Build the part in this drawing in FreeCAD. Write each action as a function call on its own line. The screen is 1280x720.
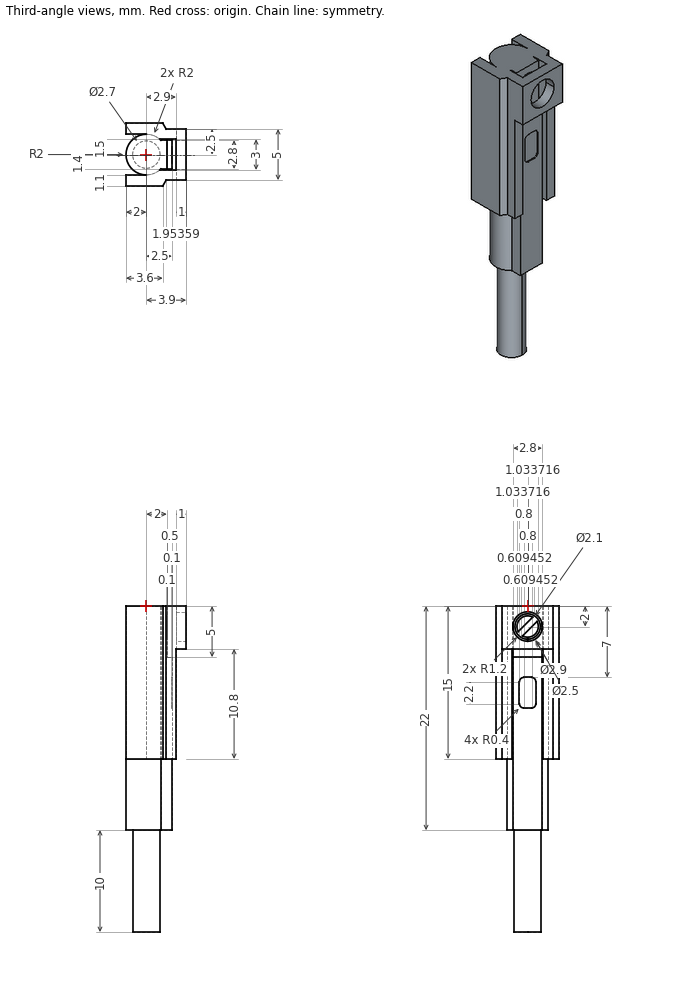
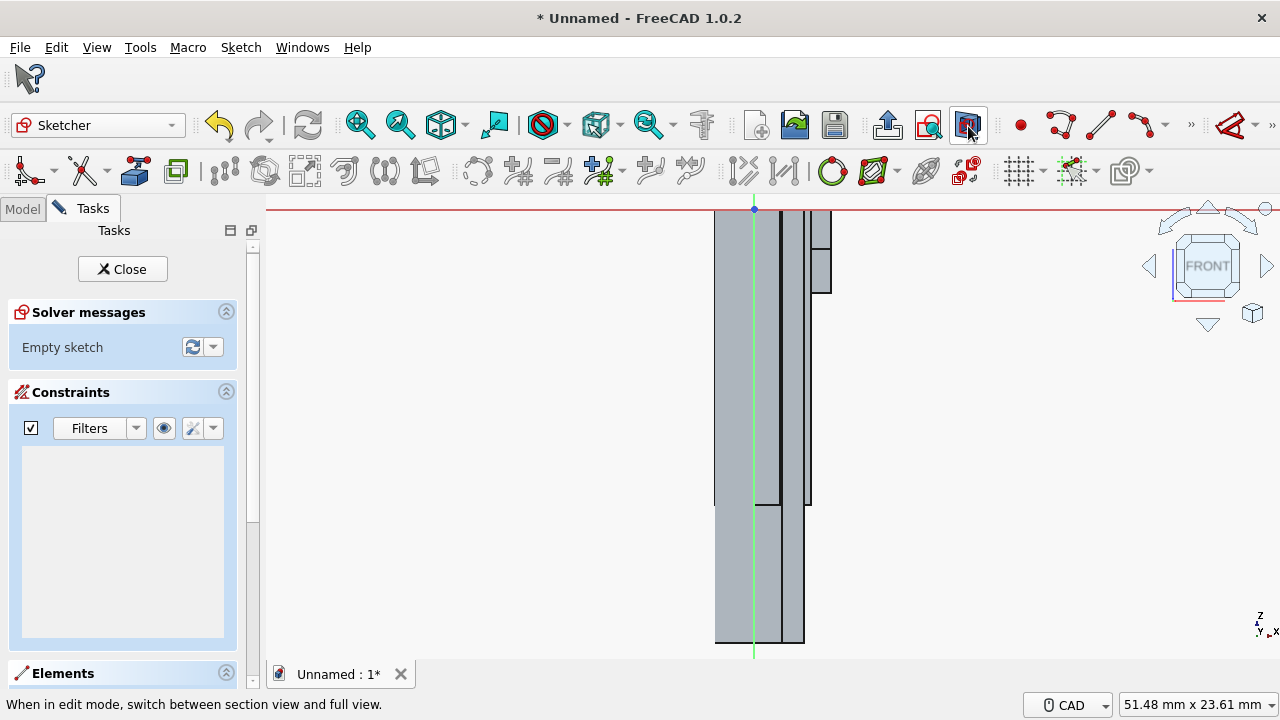
scroll(704, 426, down, 5)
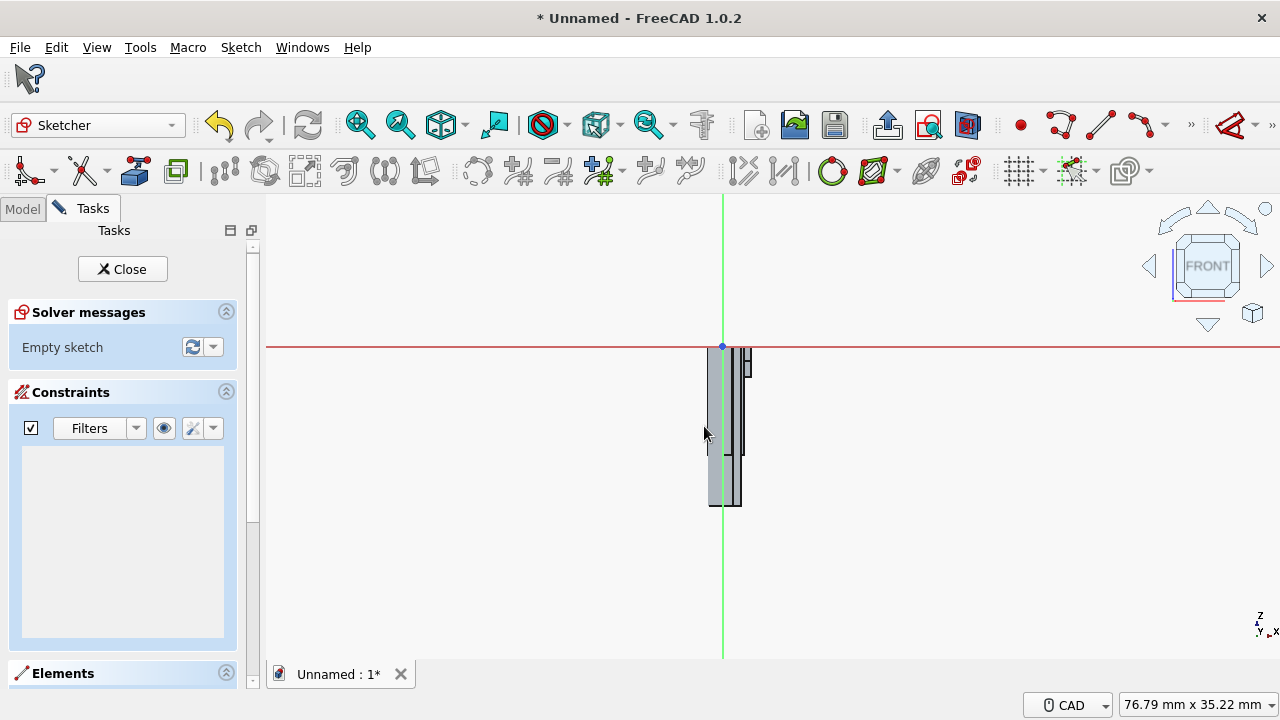
scroll(736, 355, up, 10)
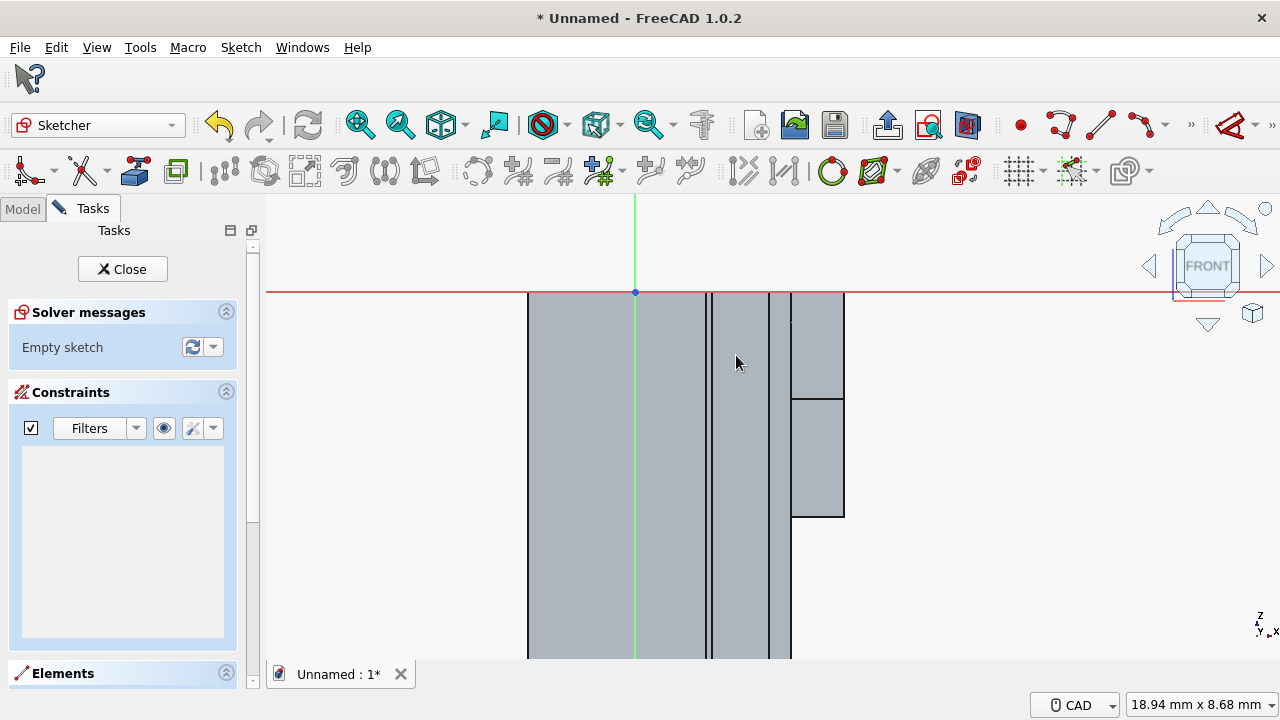
key(g)
key(r)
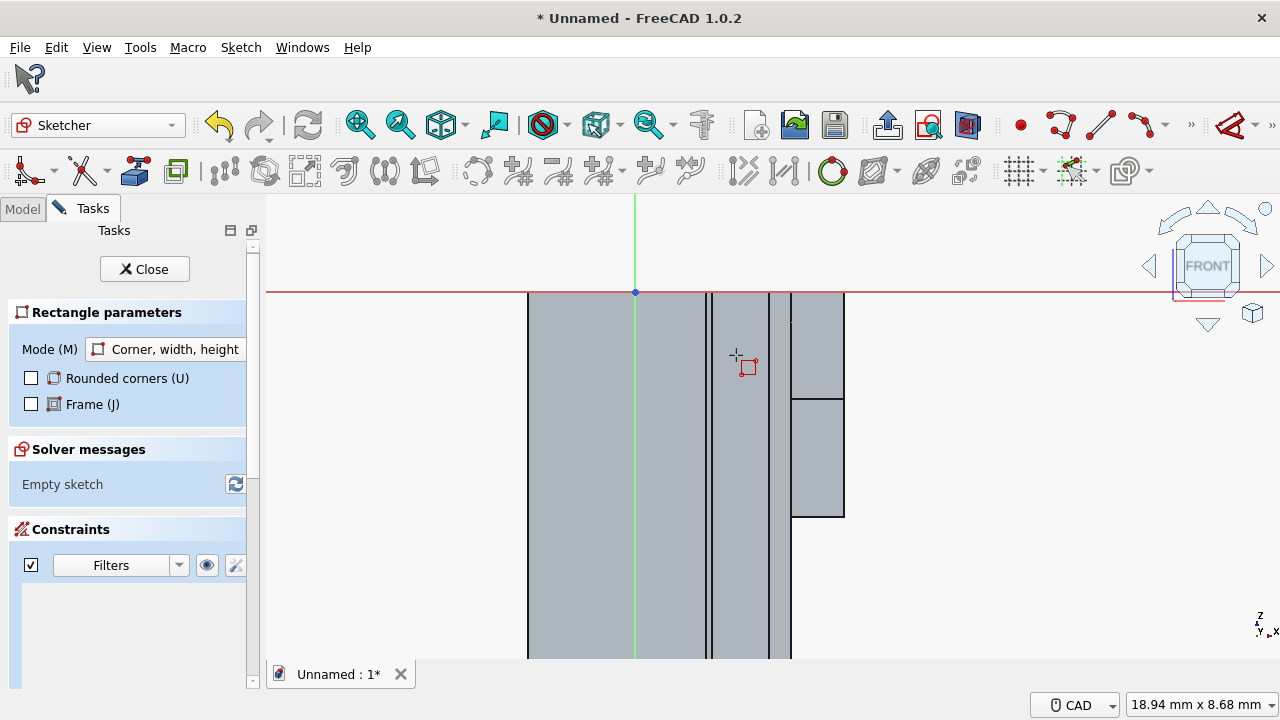
click(742, 292)
click(769, 560)
key(Escape)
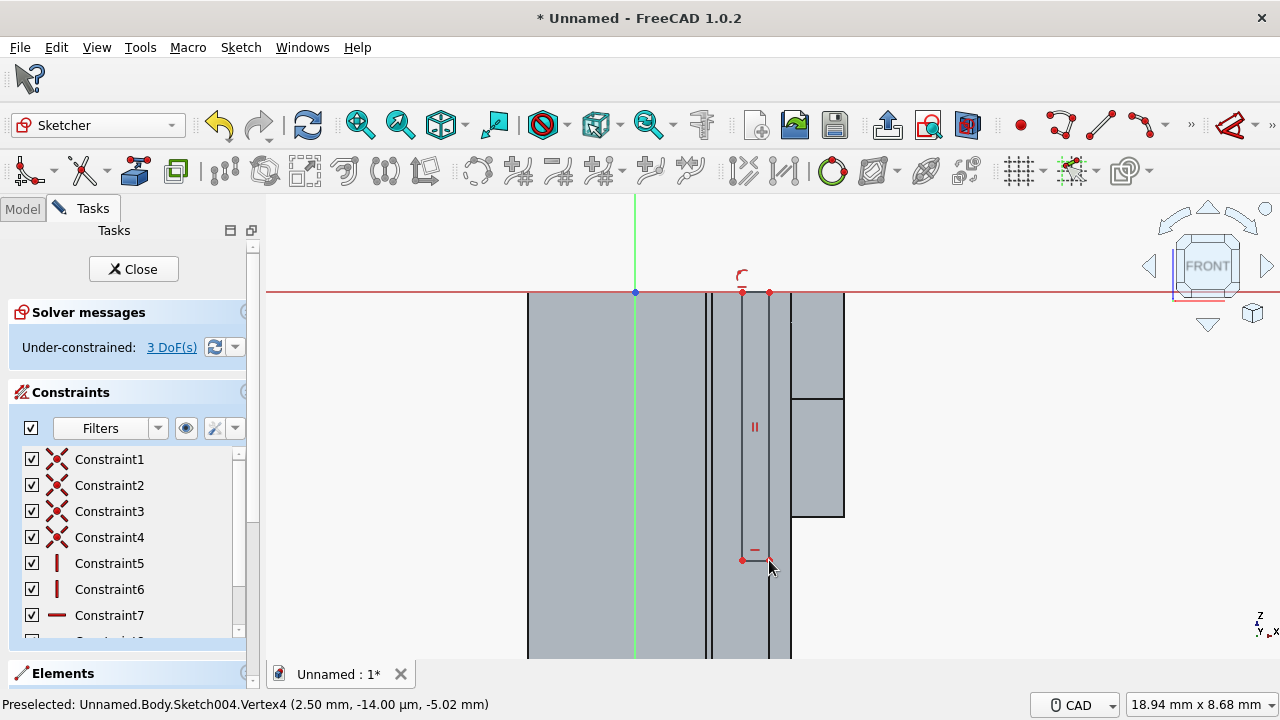
click(1230, 126)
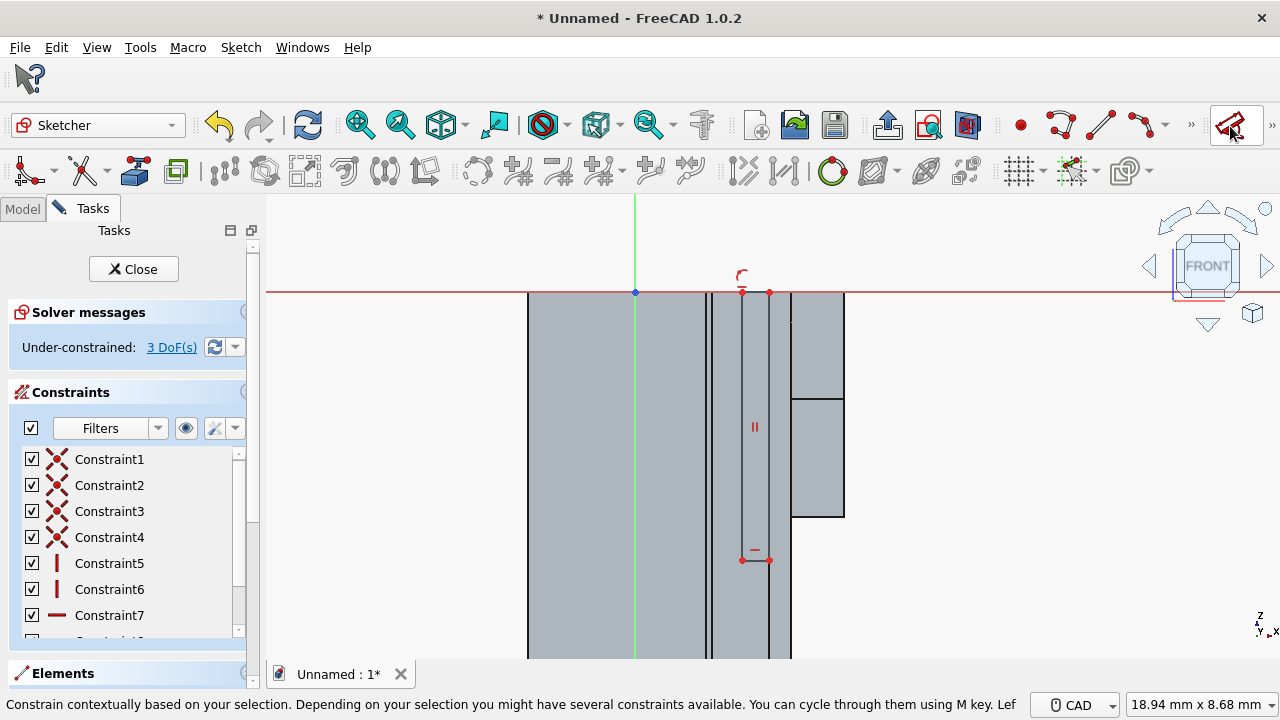
click(742, 373)
click(708, 427)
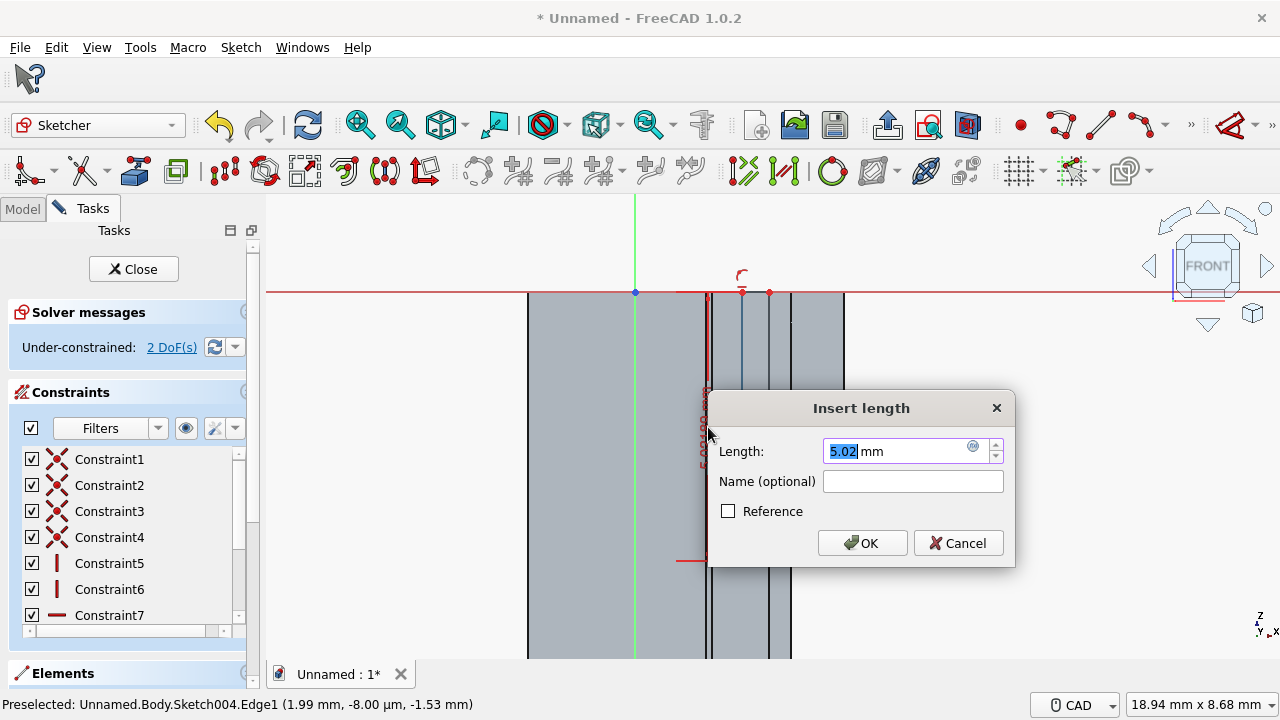
text(5)
key(Return)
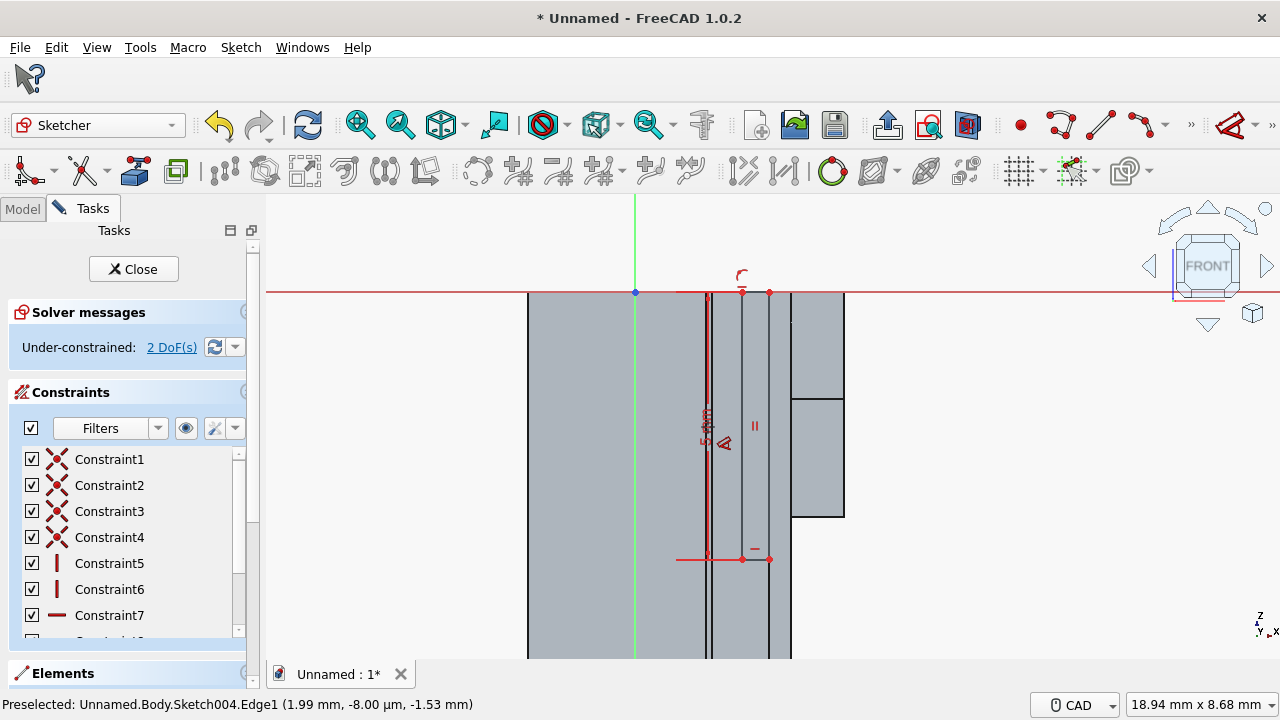
click(742, 292)
click(689, 258)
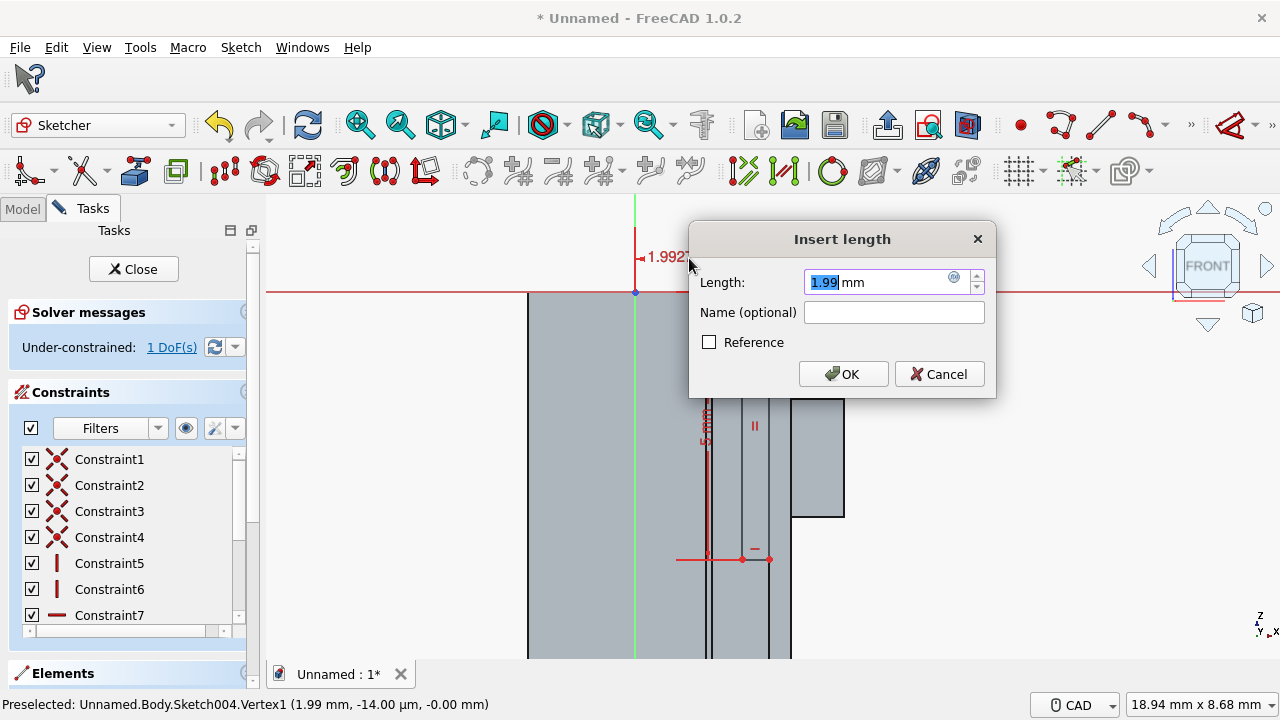
text(2)
key(Return)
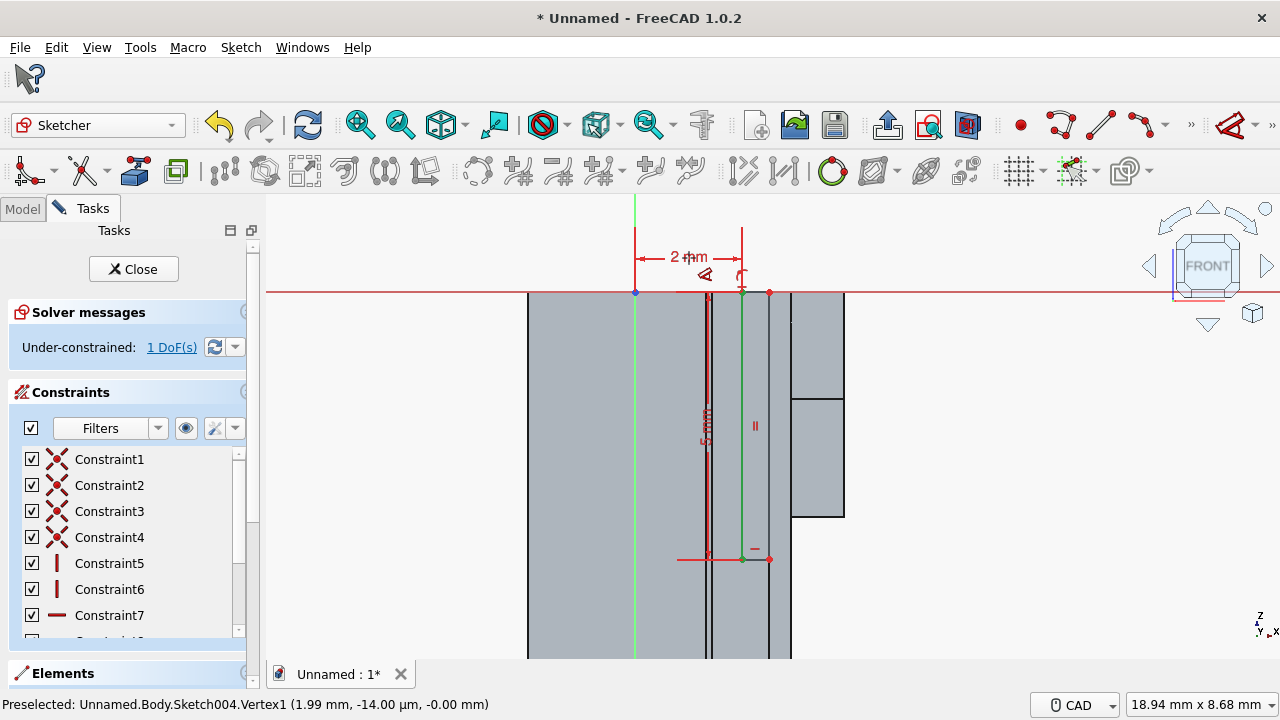
scroll(753, 560, up, 2)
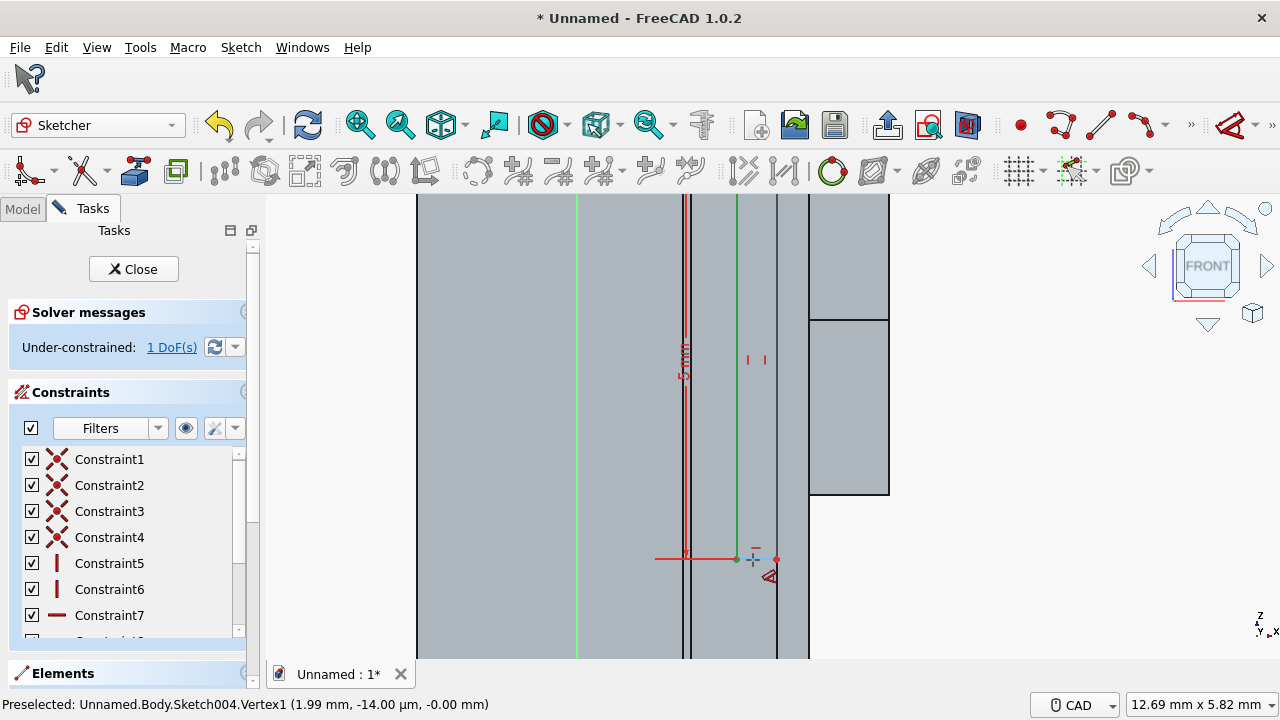
click(753, 559)
click(757, 593)